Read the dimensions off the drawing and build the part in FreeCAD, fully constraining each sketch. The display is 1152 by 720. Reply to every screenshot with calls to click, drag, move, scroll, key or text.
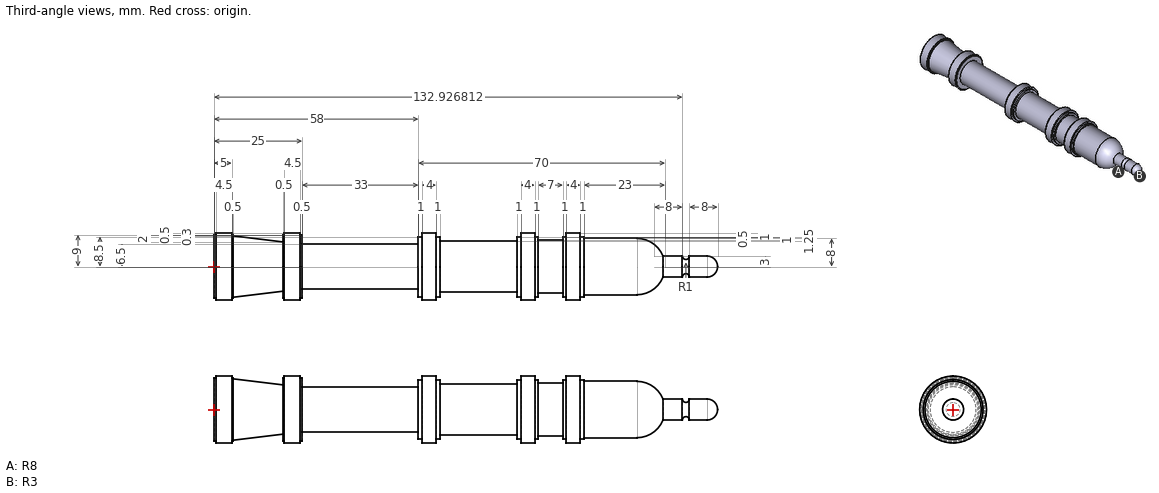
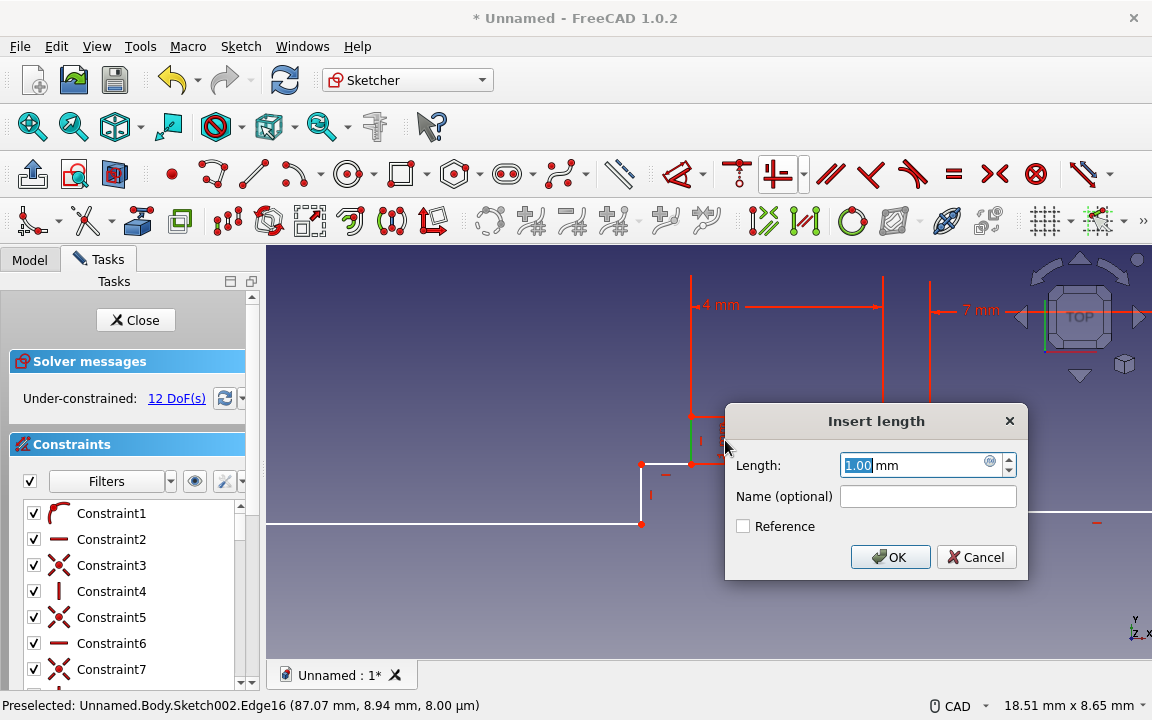
text(1)
key(Return)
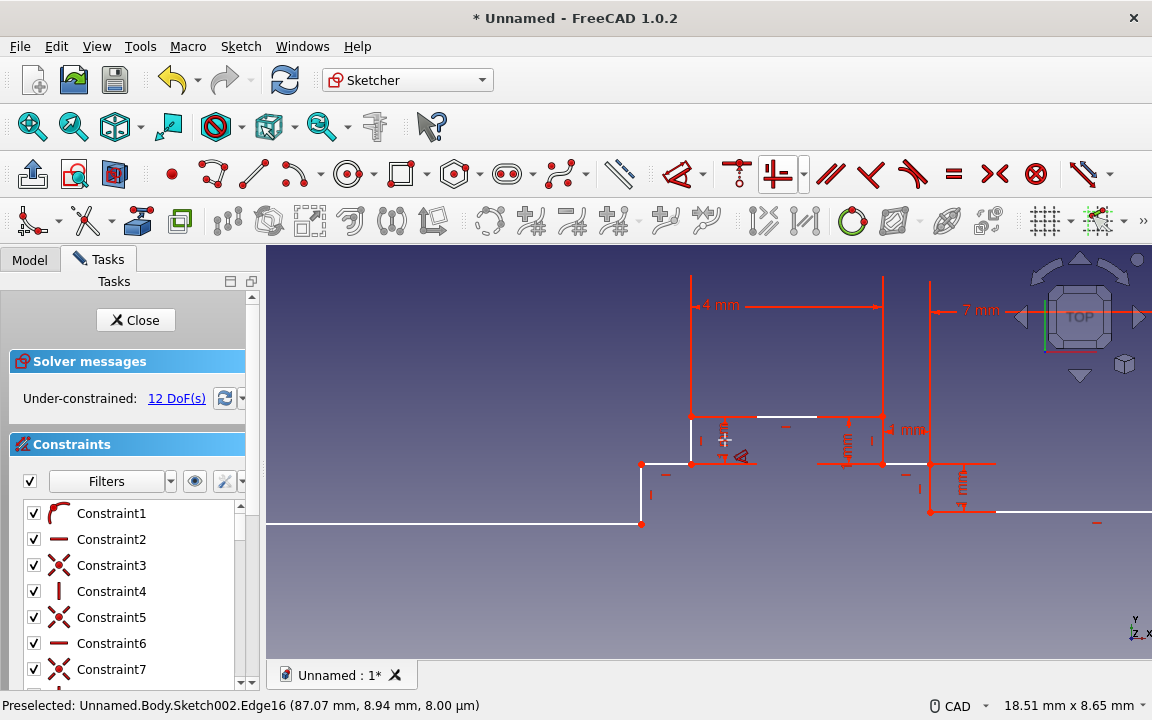
click(676, 464)
click(655, 430)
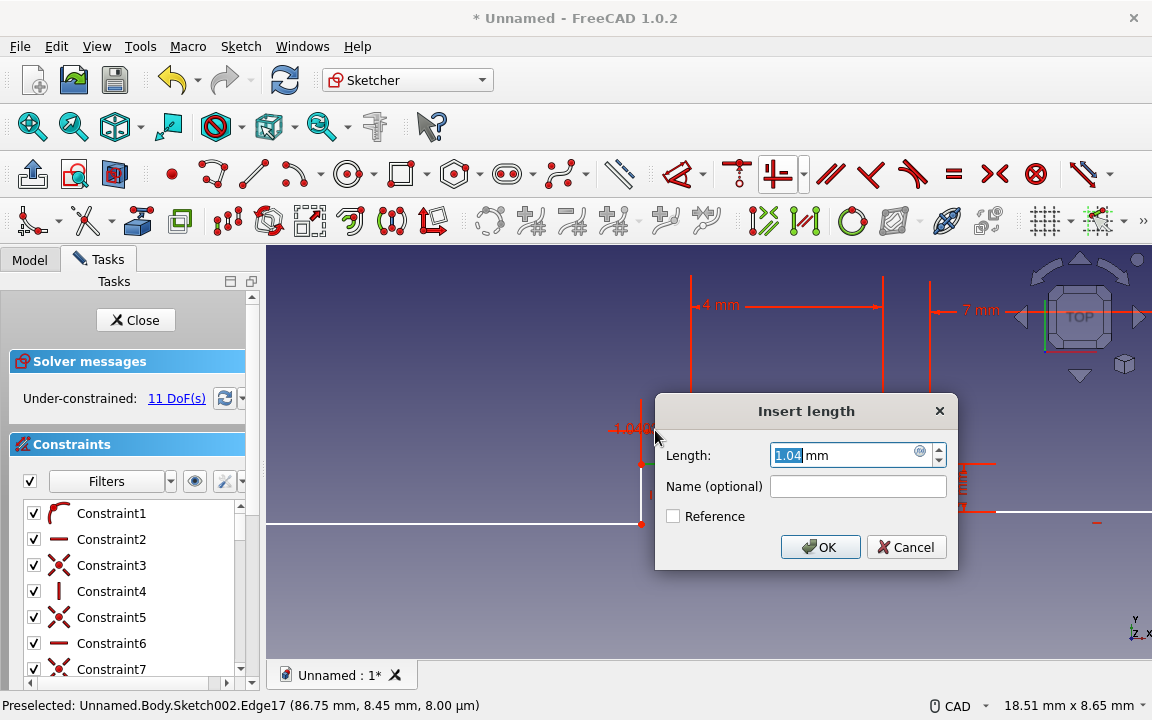
text(1)
key(Return)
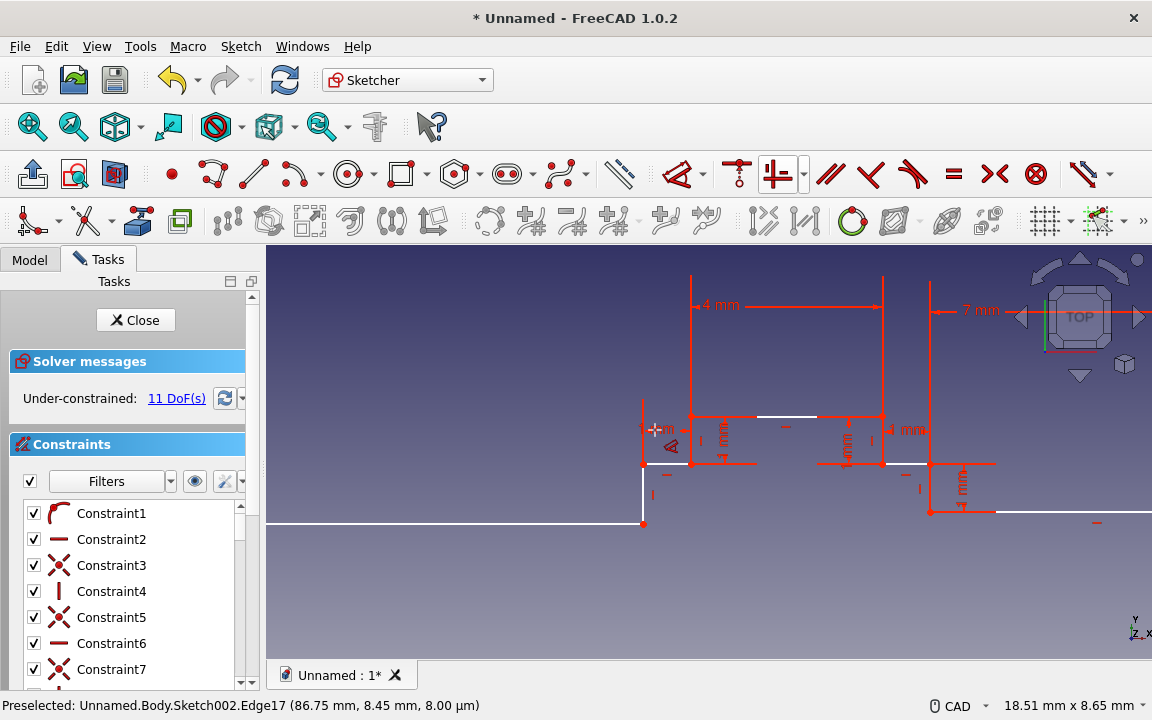
scroll(725, 437, down, 13)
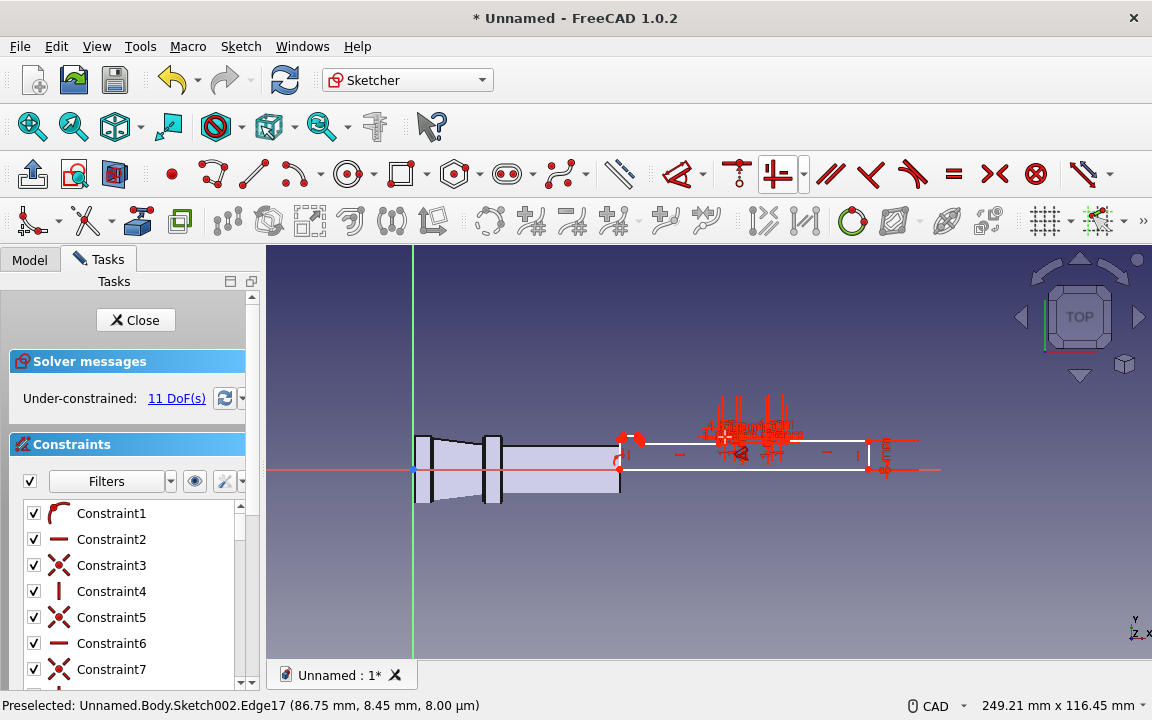
scroll(640, 440, up, 13)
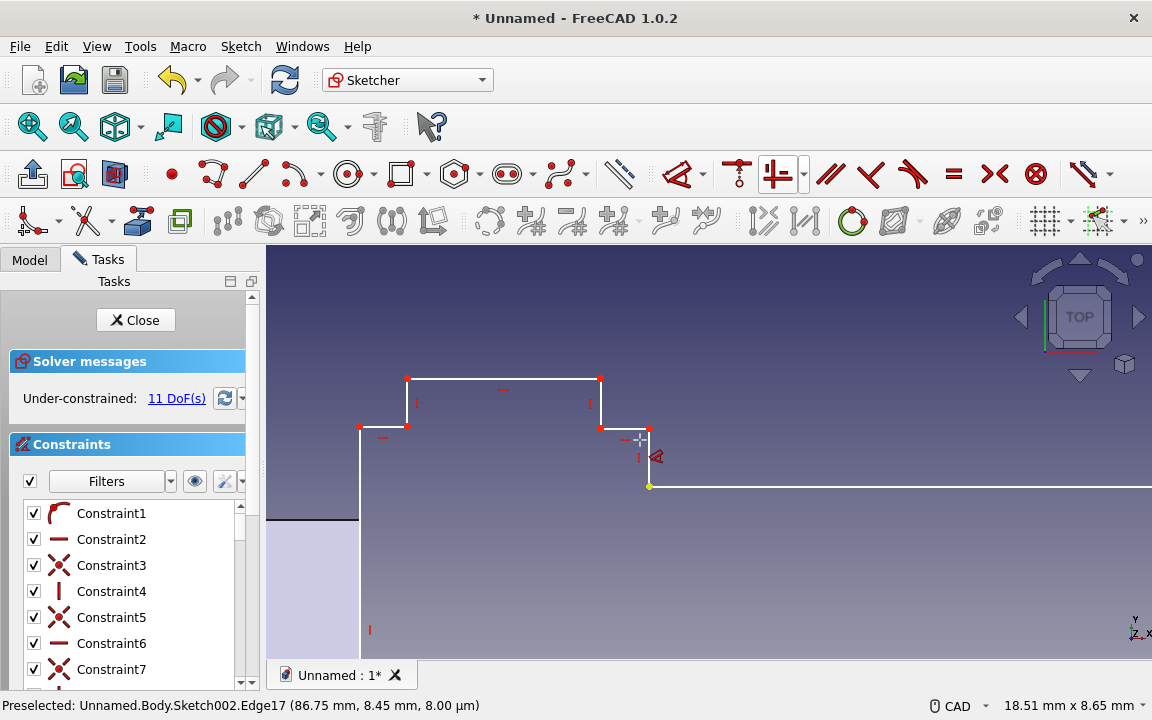
click(635, 429)
click(625, 395)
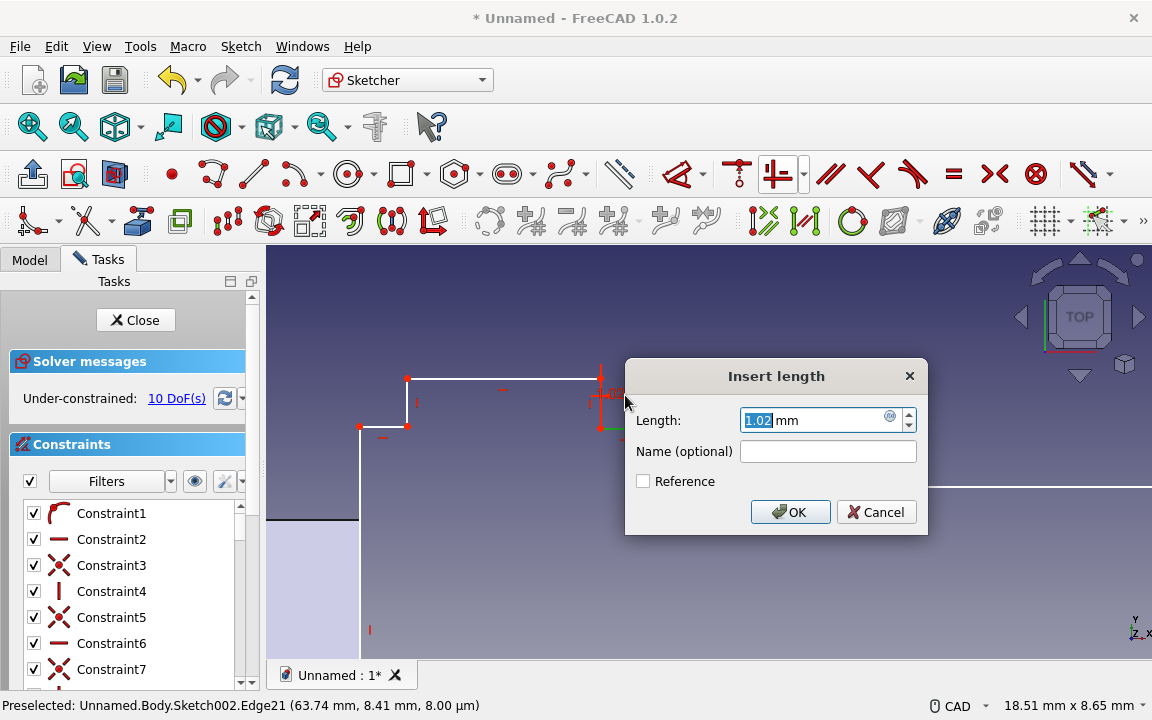
text(1)
key(Return)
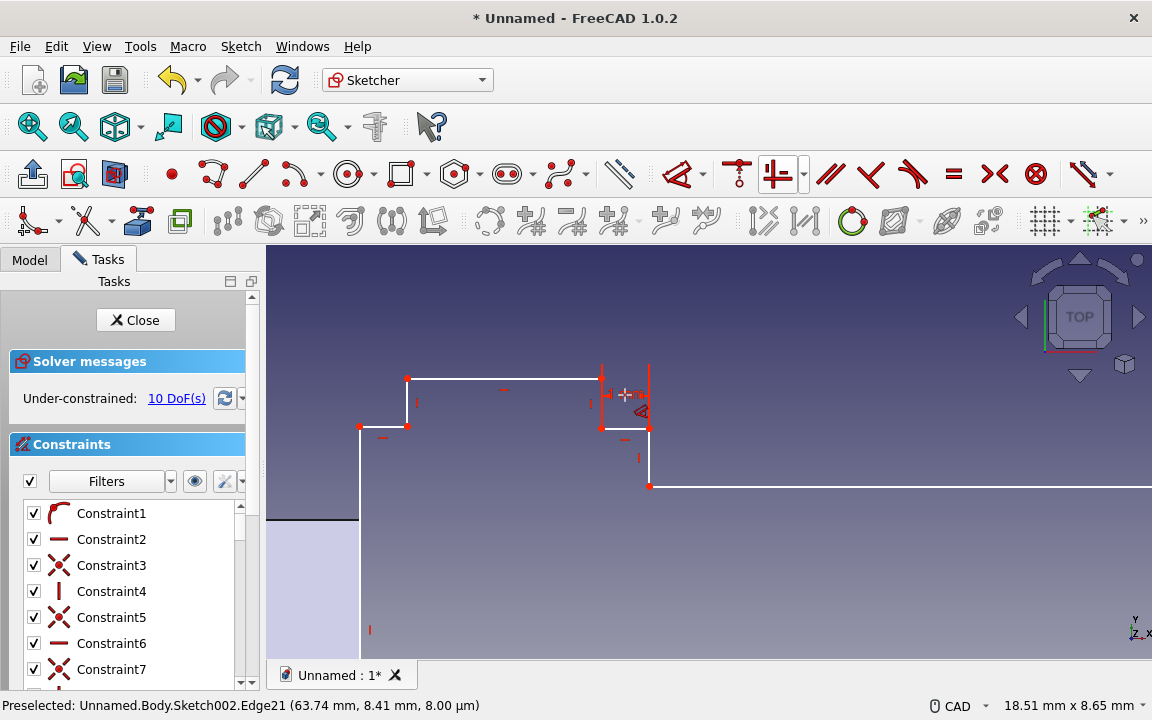
click(602, 414)
click(568, 415)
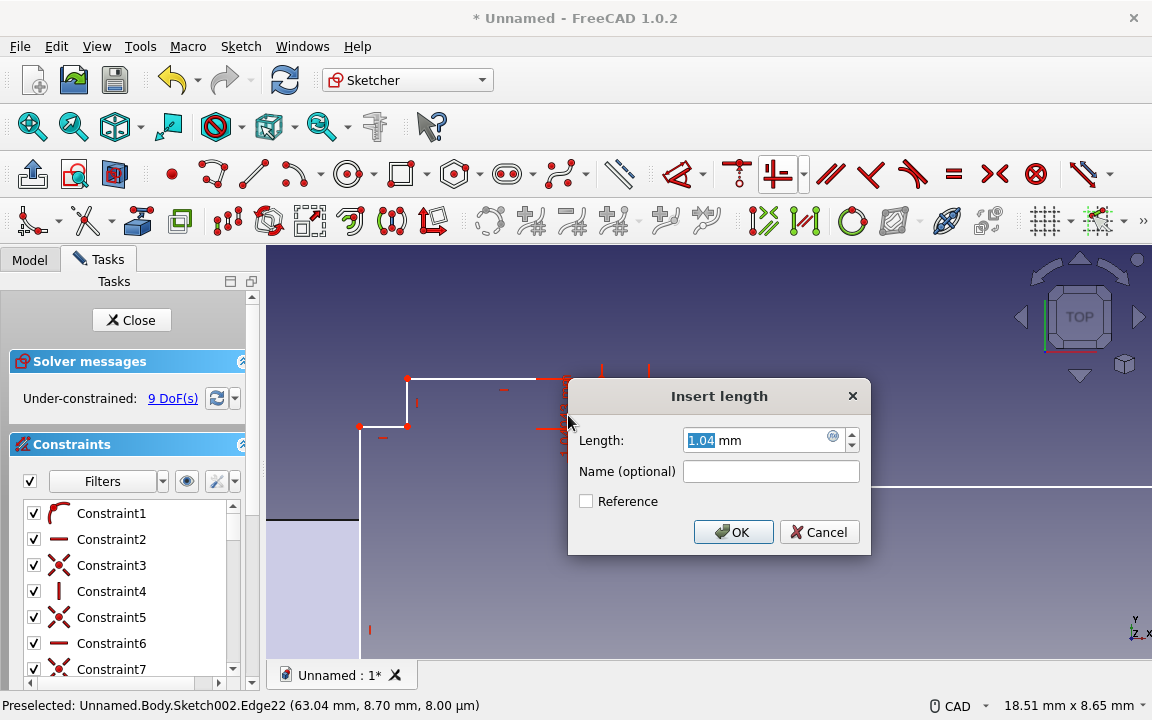
text(1)
key(Return)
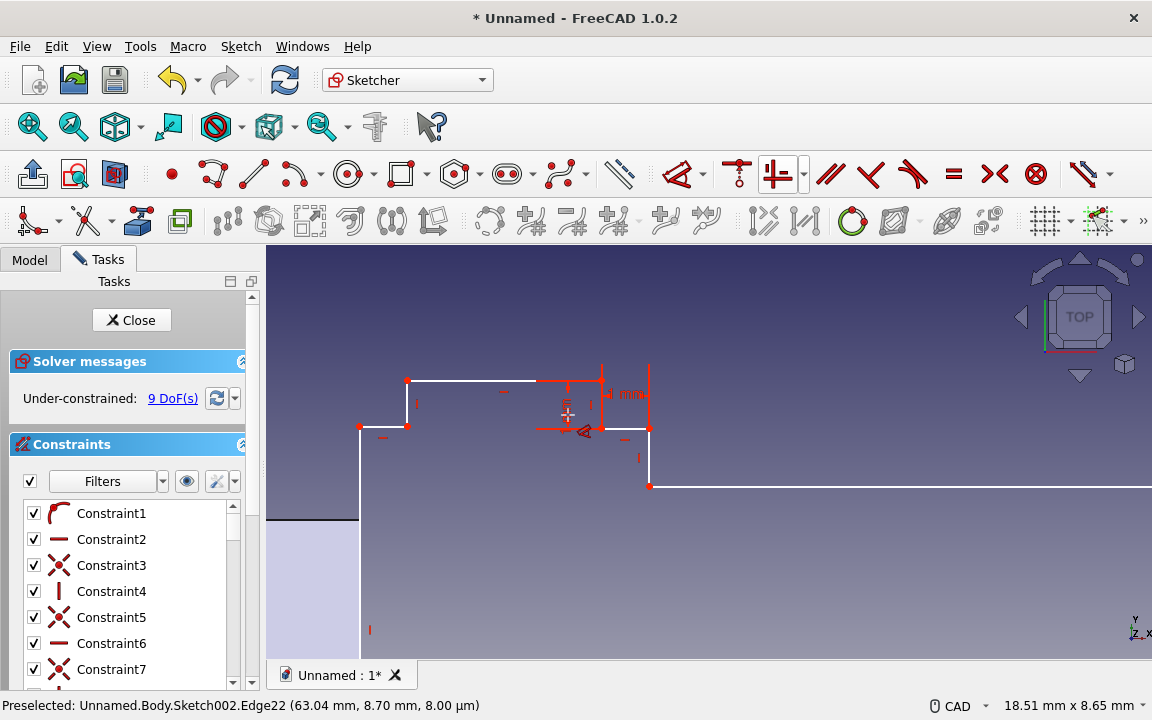
scroll(640, 440, down, 13)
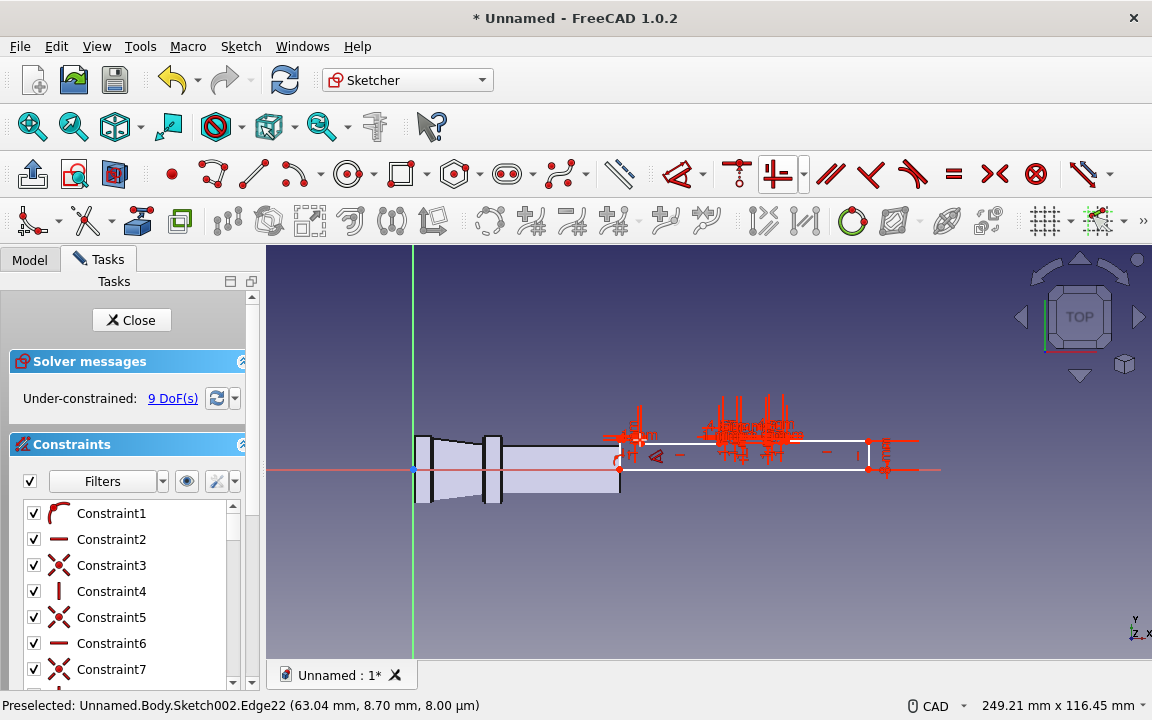
scroll(633, 436, up, 6)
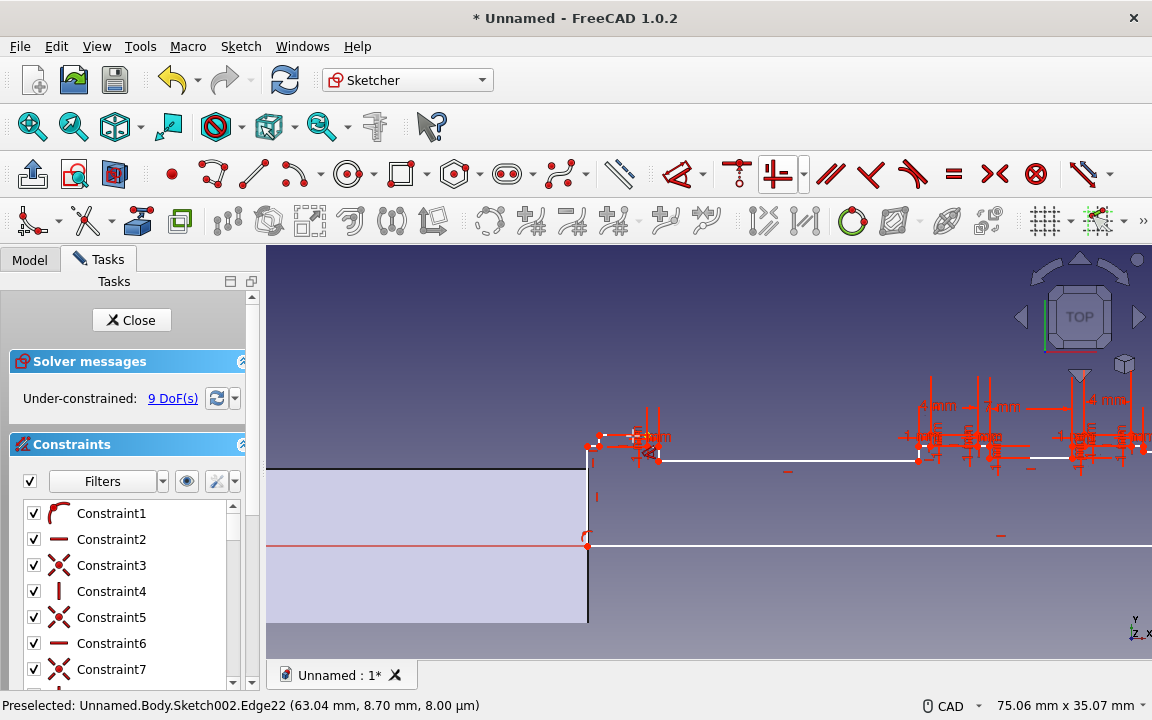
click(633, 435)
click(623, 401)